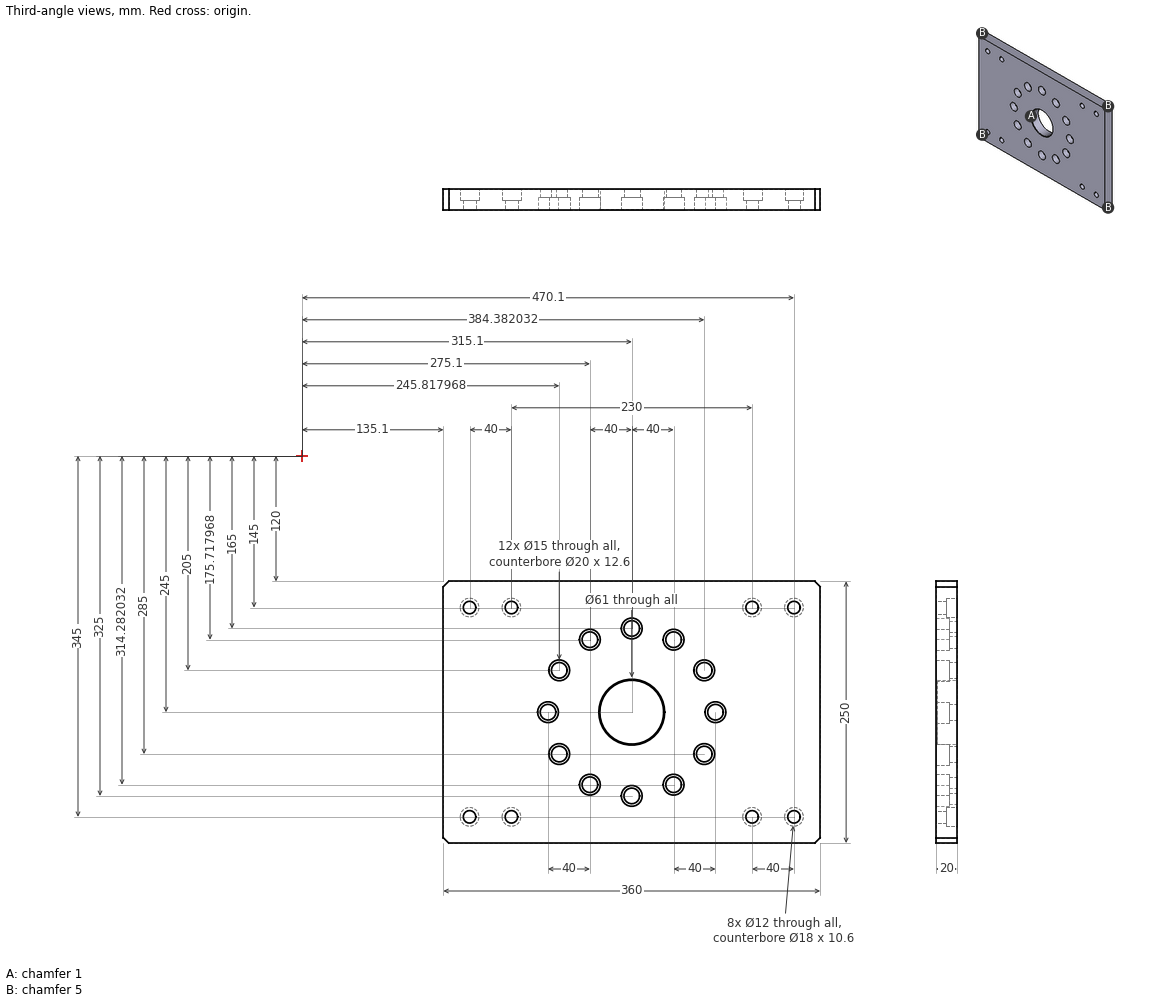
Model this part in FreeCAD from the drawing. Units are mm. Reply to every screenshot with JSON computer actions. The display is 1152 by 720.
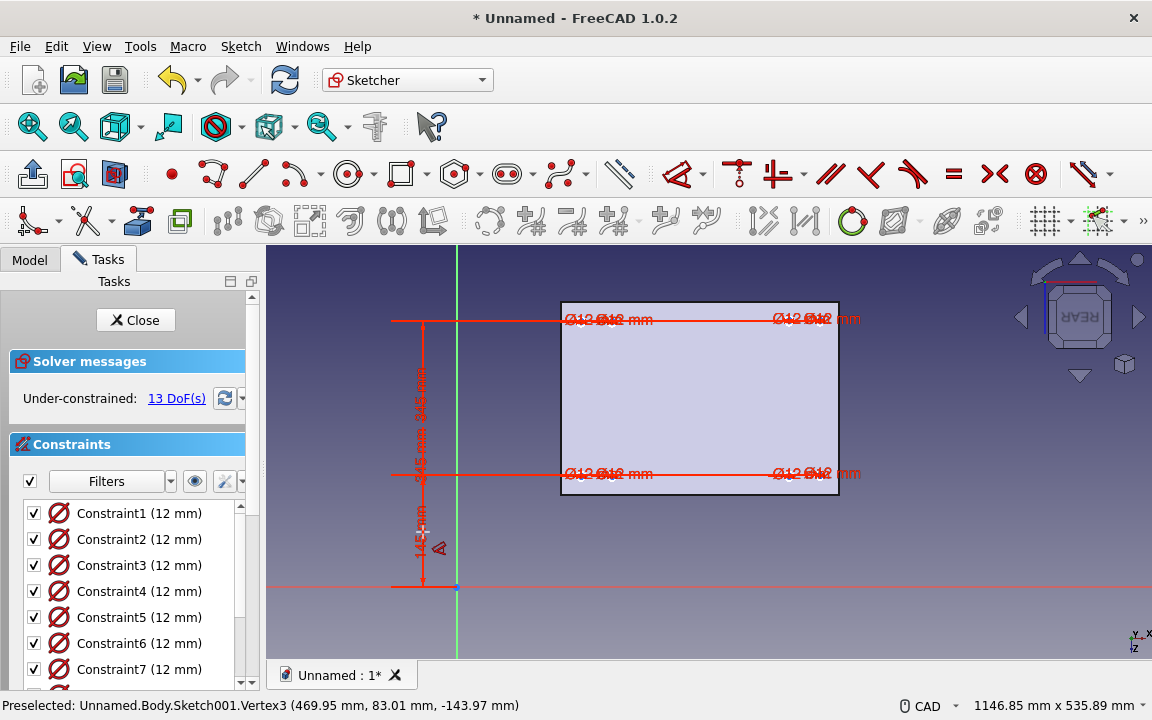
{"action": "left_click", "coordinate": [789, 476]}
{"action": "left_click", "coordinate": [423, 506]}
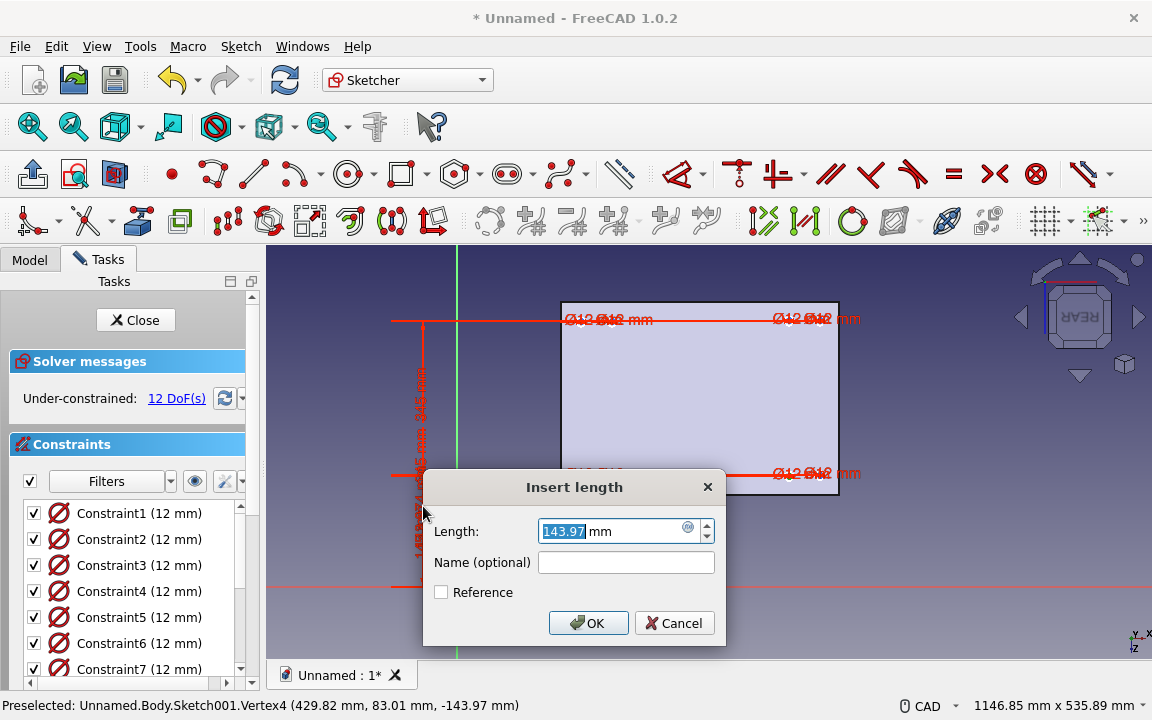
{"action": "type", "text": "145"}
{"action": "key", "text": "Return"}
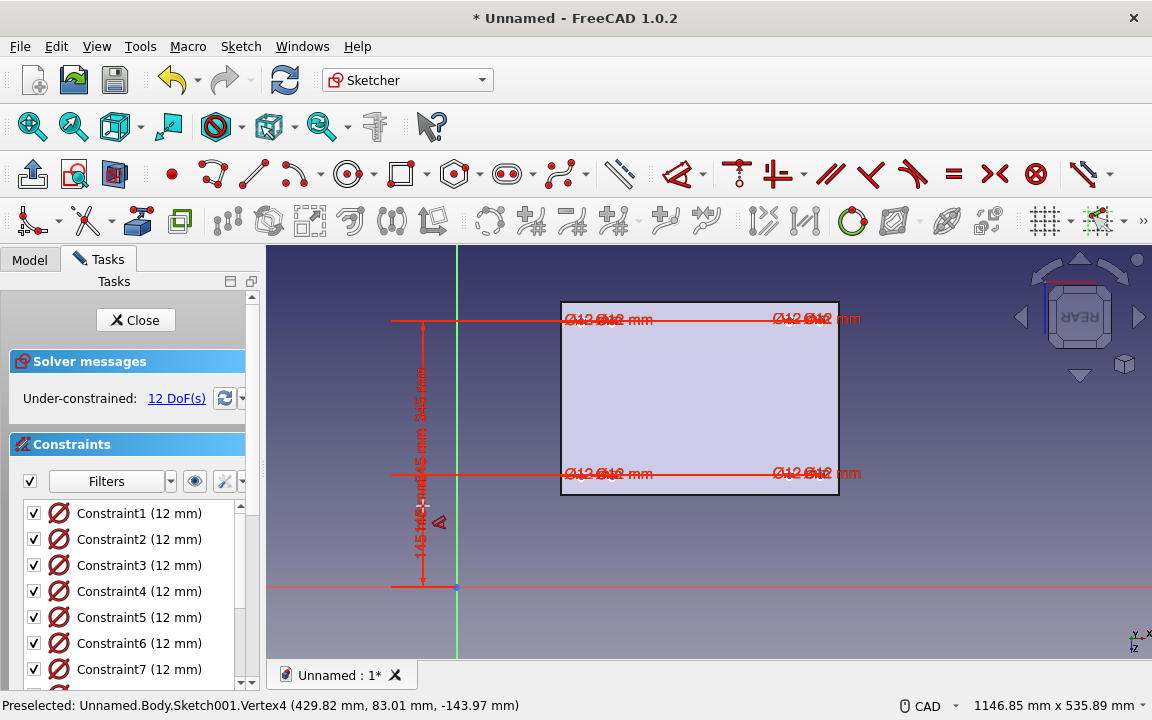
{"action": "left_click", "coordinate": [612, 476]}
{"action": "left_click", "coordinate": [423, 557]}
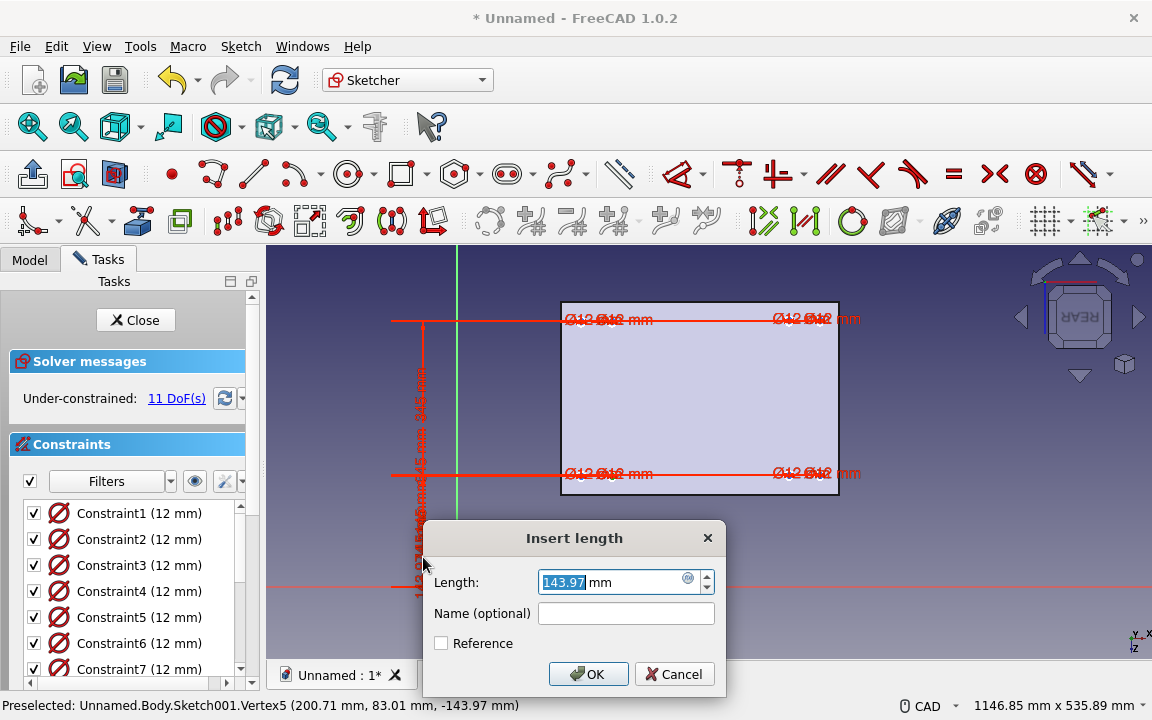
{"action": "type", "text": "145"}
{"action": "key", "text": "Return"}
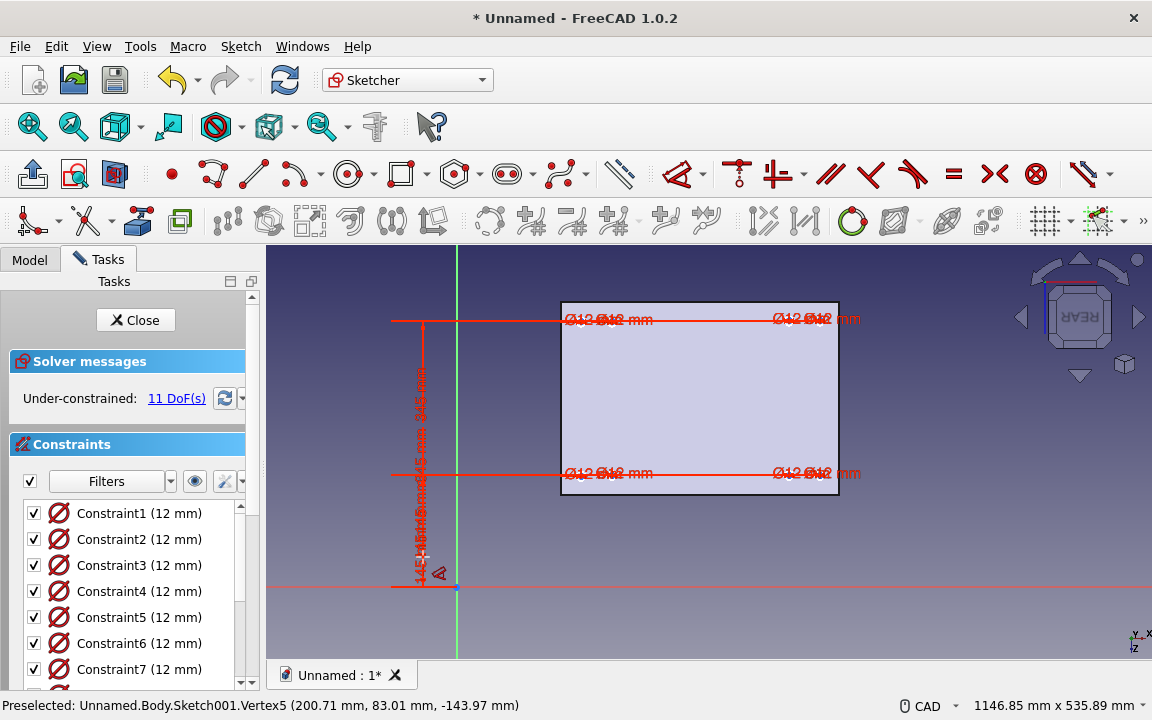
{"action": "left_click", "coordinate": [612, 322]}
{"action": "left_click", "coordinate": [423, 362]}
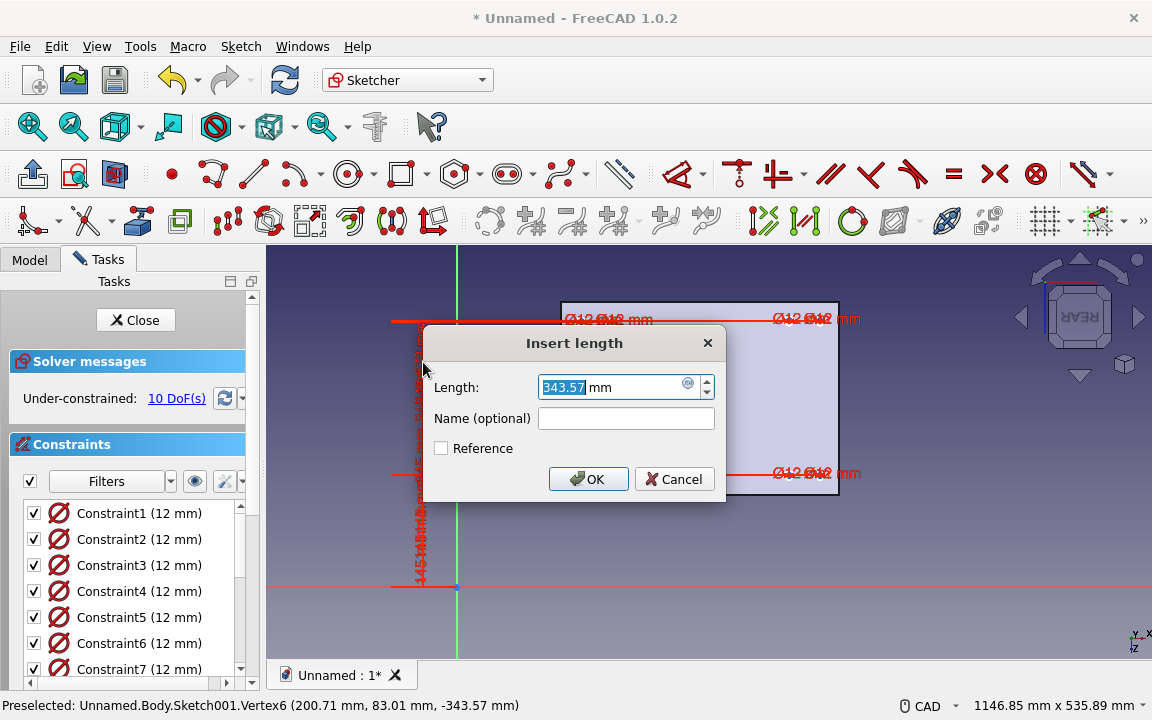
{"action": "type", "text": "345"}
{"action": "key", "text": "Return"}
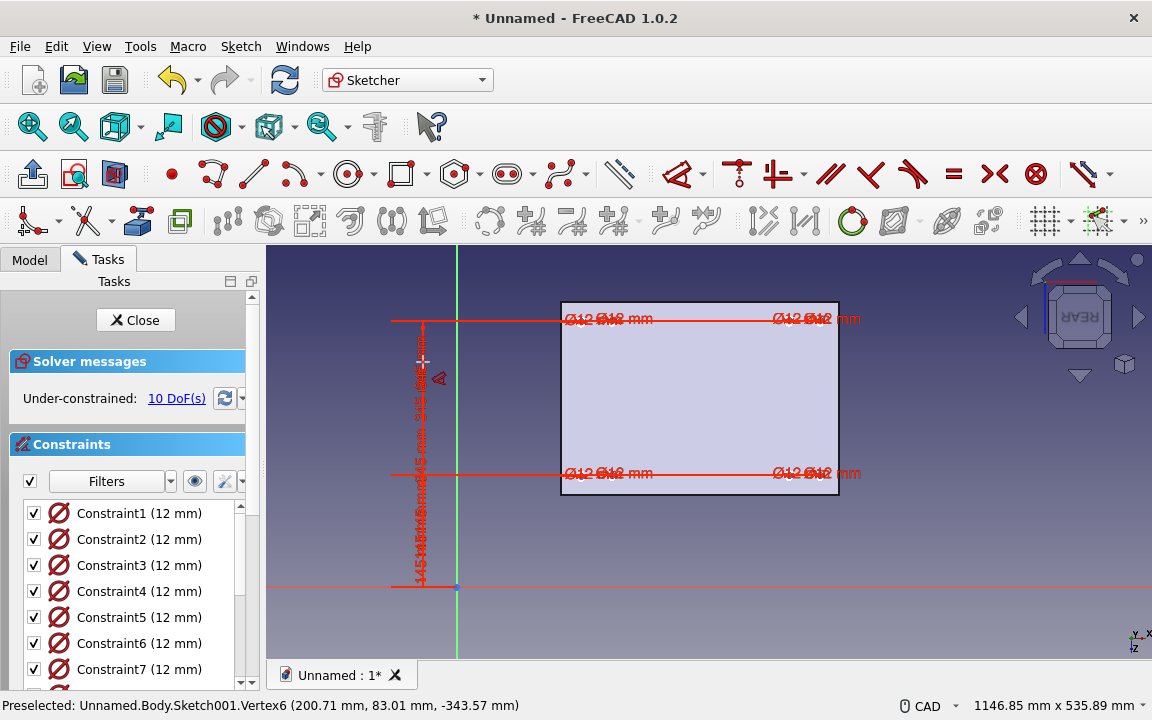
{"action": "left_click", "coordinate": [581, 476]}
{"action": "left_click", "coordinate": [615, 532]}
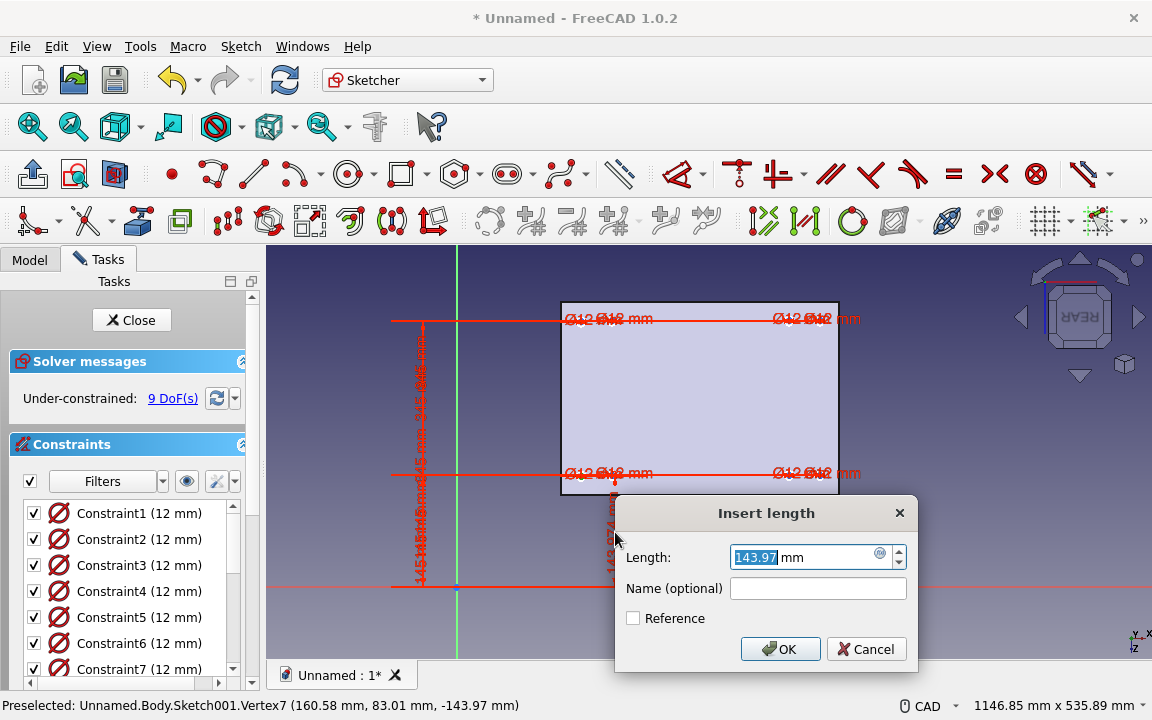
{"action": "type", "text": "145"}
{"action": "key", "text": "Return"}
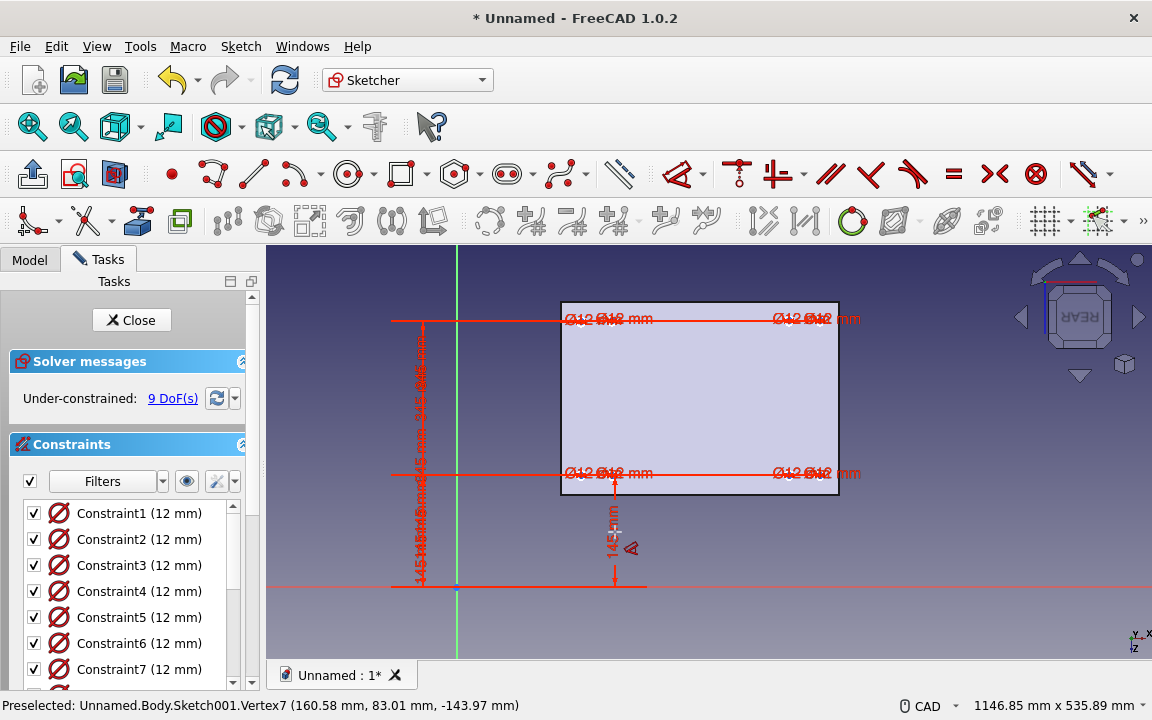
{"action": "left_click", "coordinate": [581, 322]}
{"action": "left_click", "coordinate": [615, 455]}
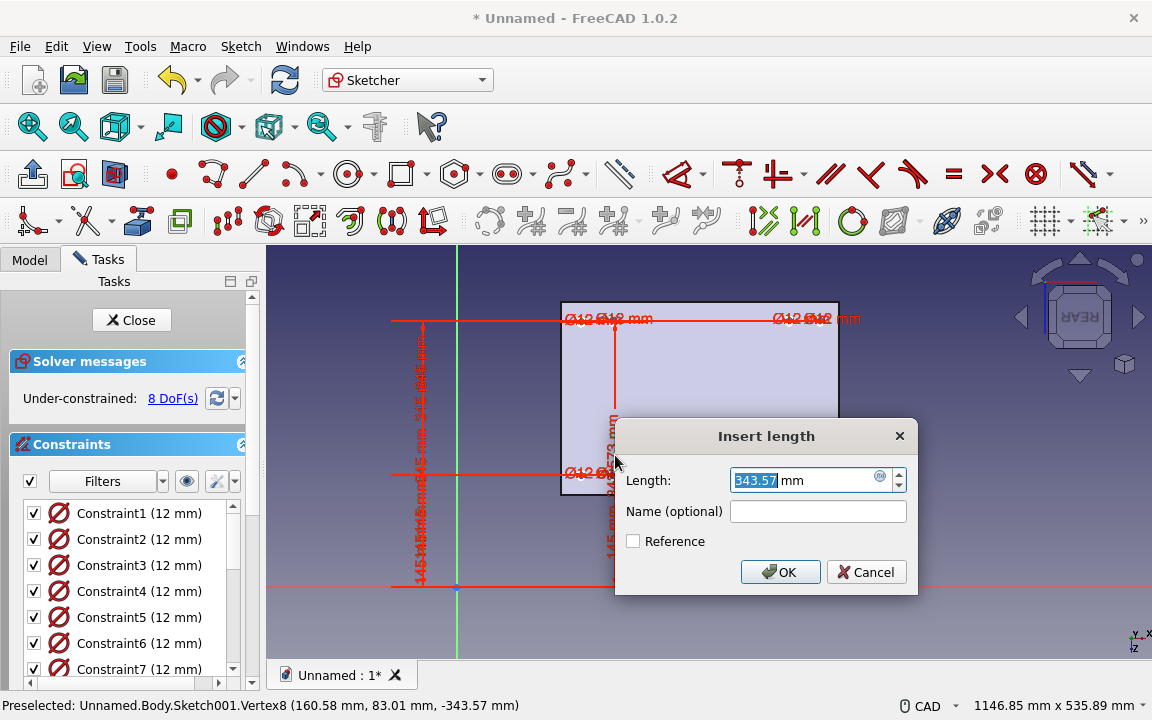
{"action": "type", "text": "345"}
{"action": "key", "text": "Return"}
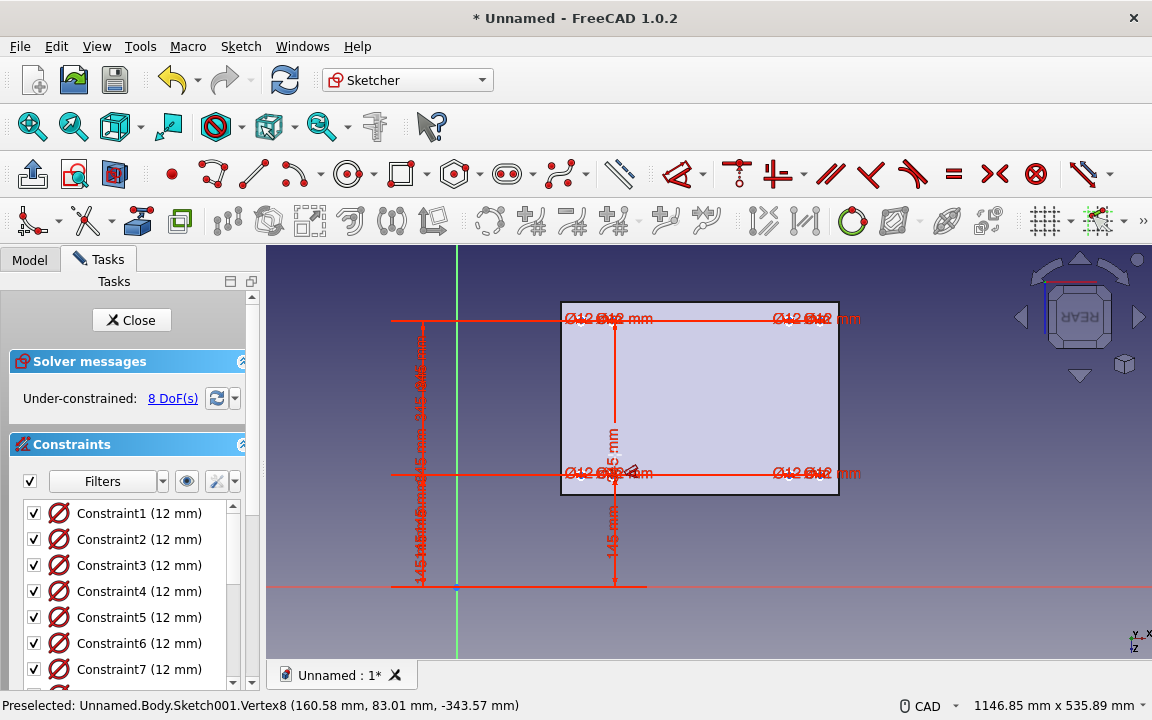
{"action": "scroll", "coordinate": [820, 321], "scroll_direction": "up", "scroll_amount": 2}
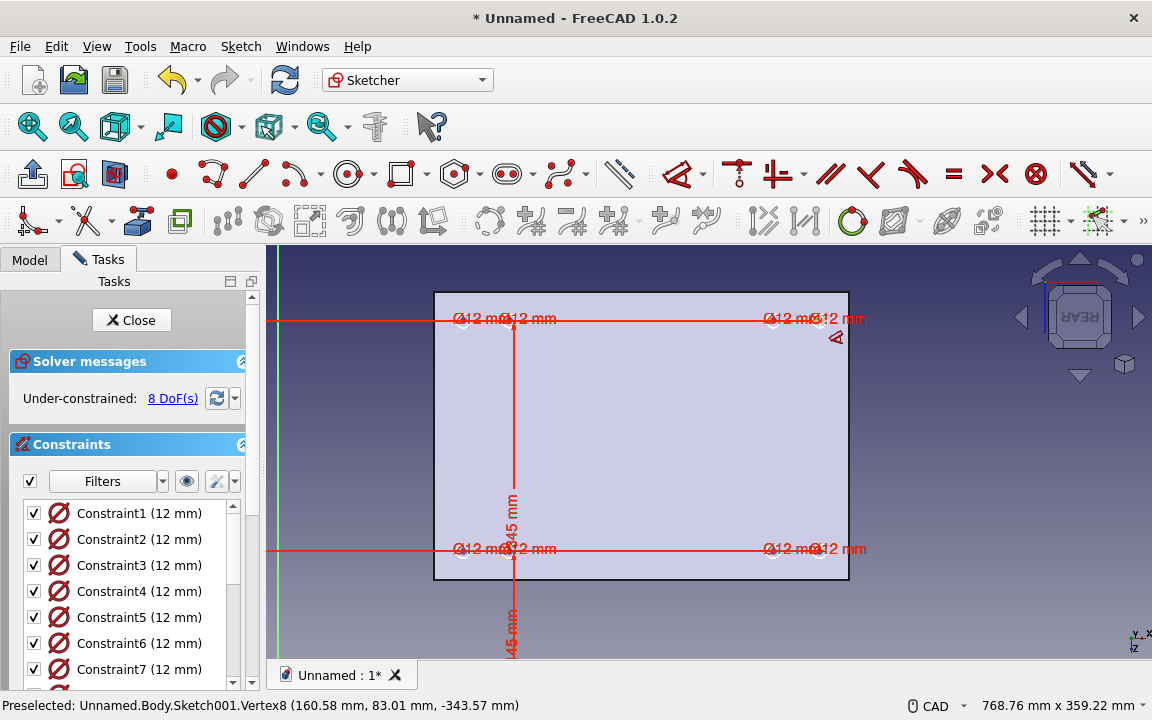
{"action": "left_click", "coordinate": [820, 321]}